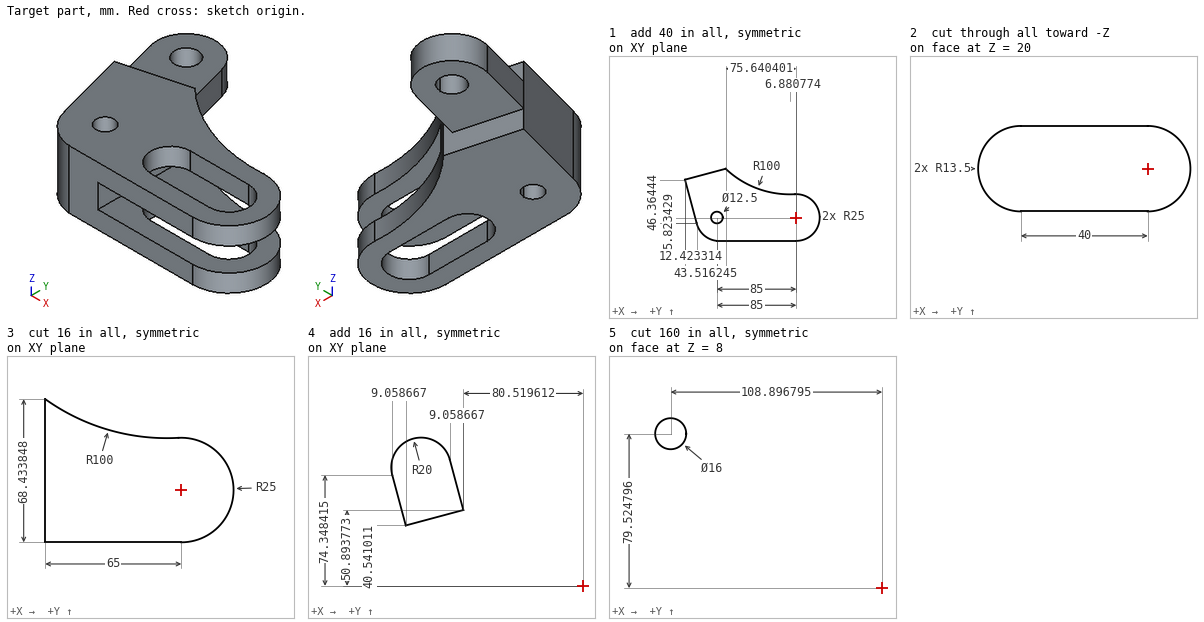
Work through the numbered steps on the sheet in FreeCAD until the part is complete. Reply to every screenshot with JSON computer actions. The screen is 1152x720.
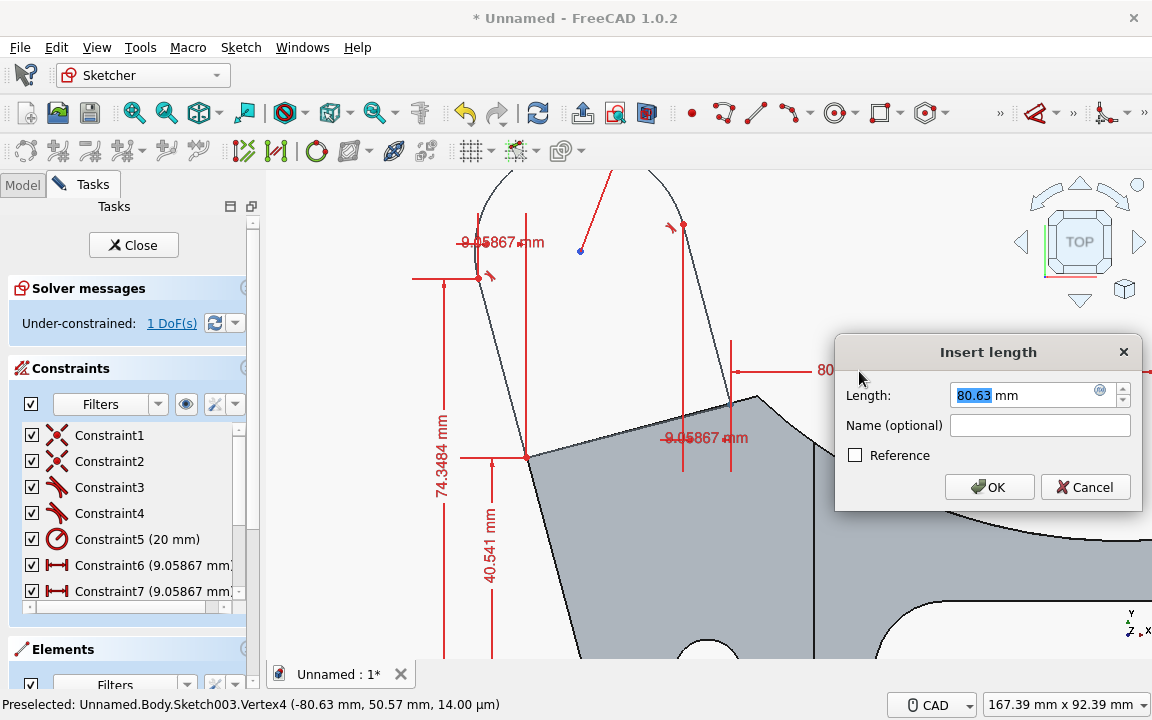
{"action": "type", "text": "80.519612"}
{"action": "key", "text": "Return"}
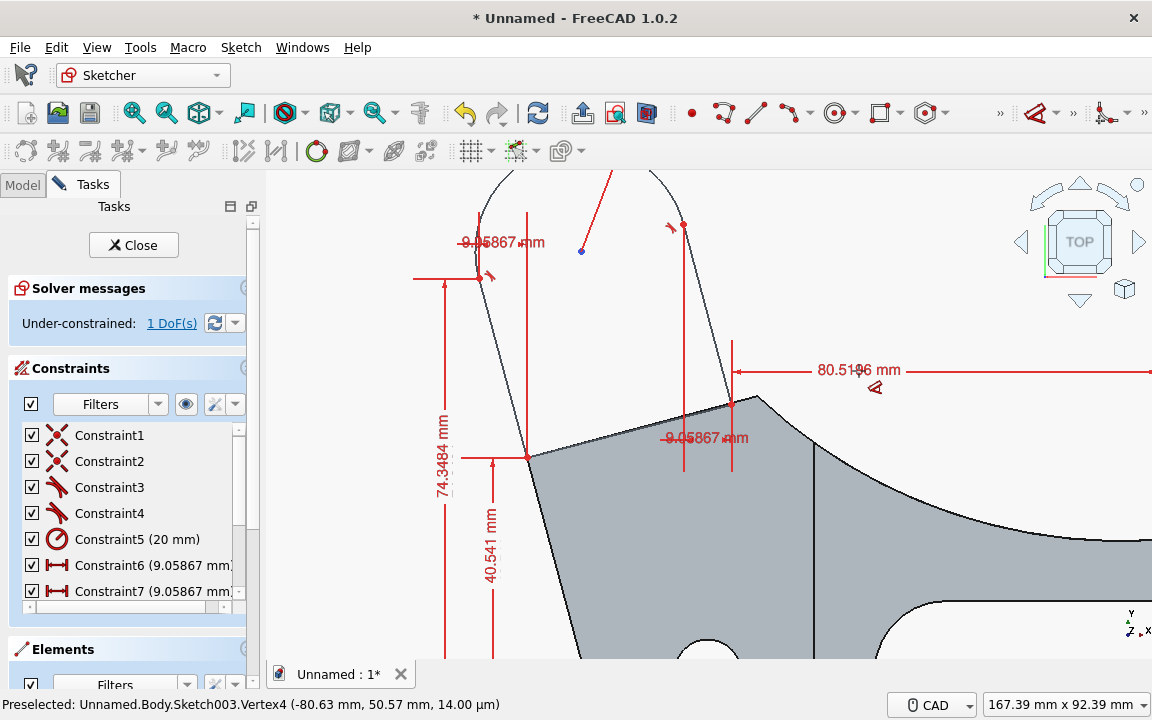
{"action": "left_click", "coordinate": [732, 405]}
{"action": "left_click", "coordinate": [698, 518]}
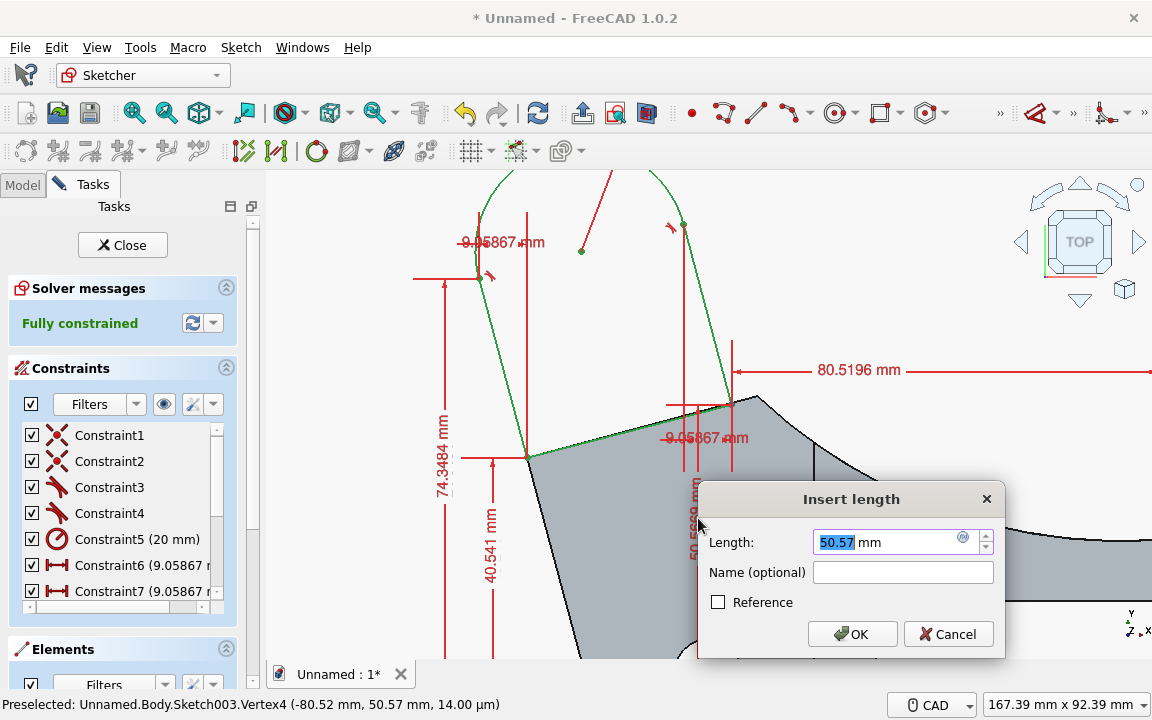
{"action": "type", "text": "50.893773"}
{"action": "key", "text": "Return"}
{"action": "key", "text": "Escape"}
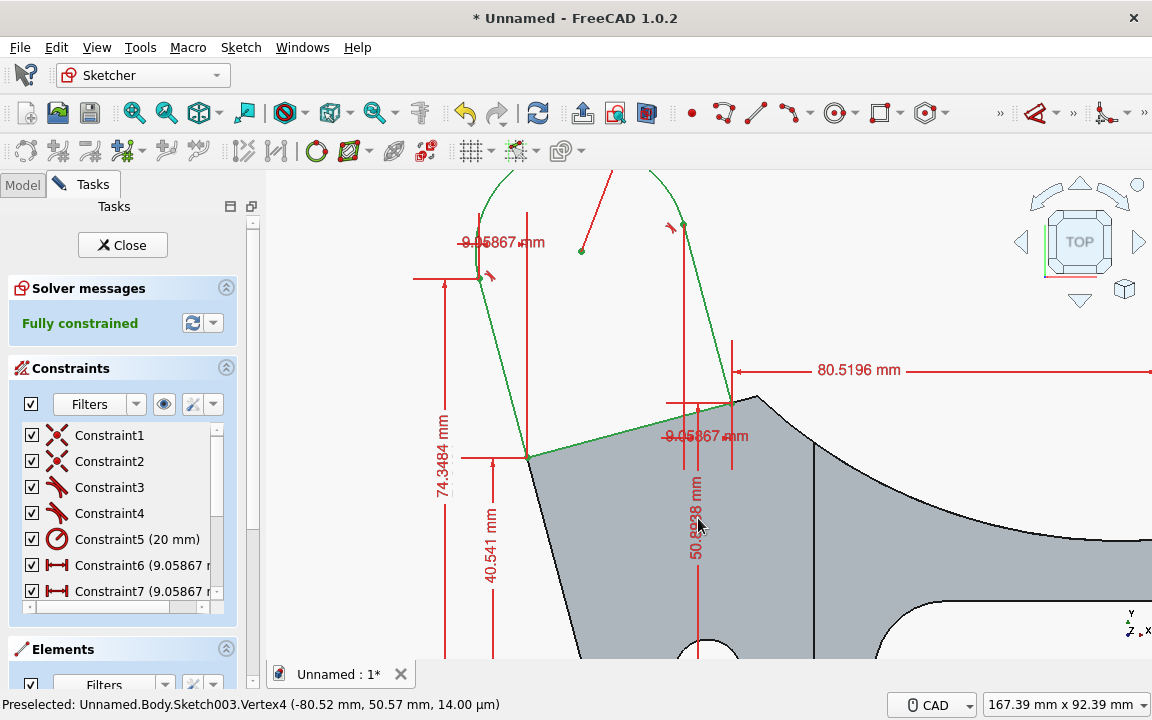
{"action": "left_click", "coordinate": [123, 245]}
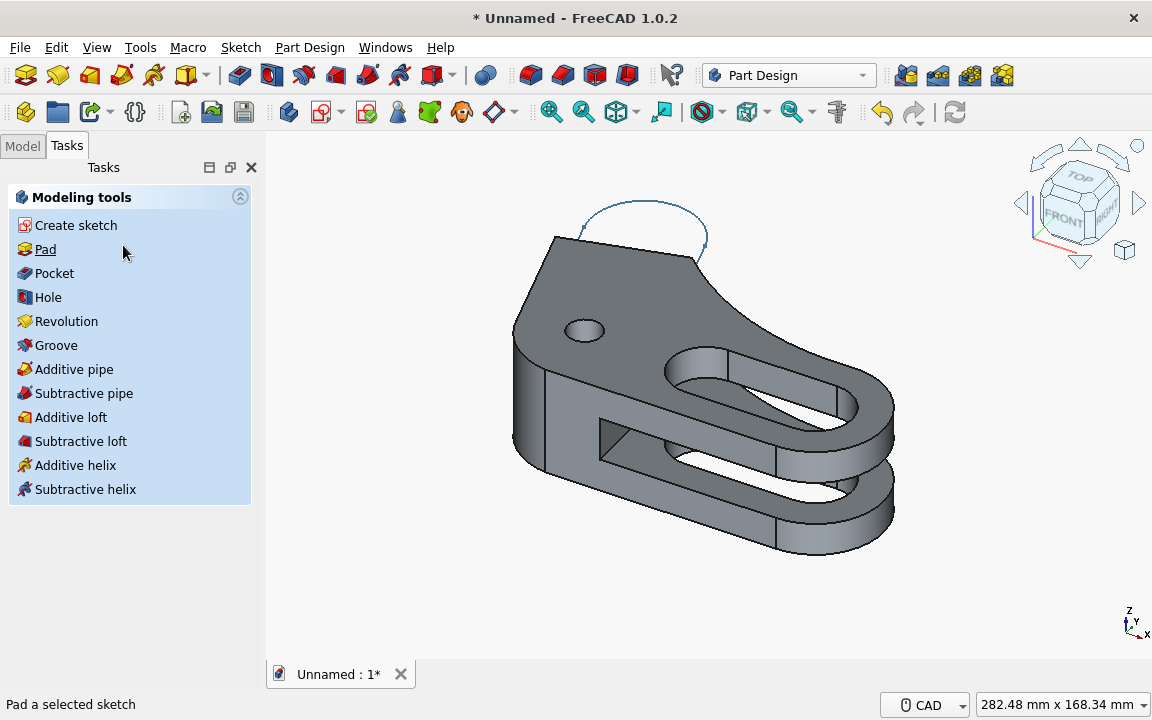
{"action": "left_click", "coordinate": [26, 76]}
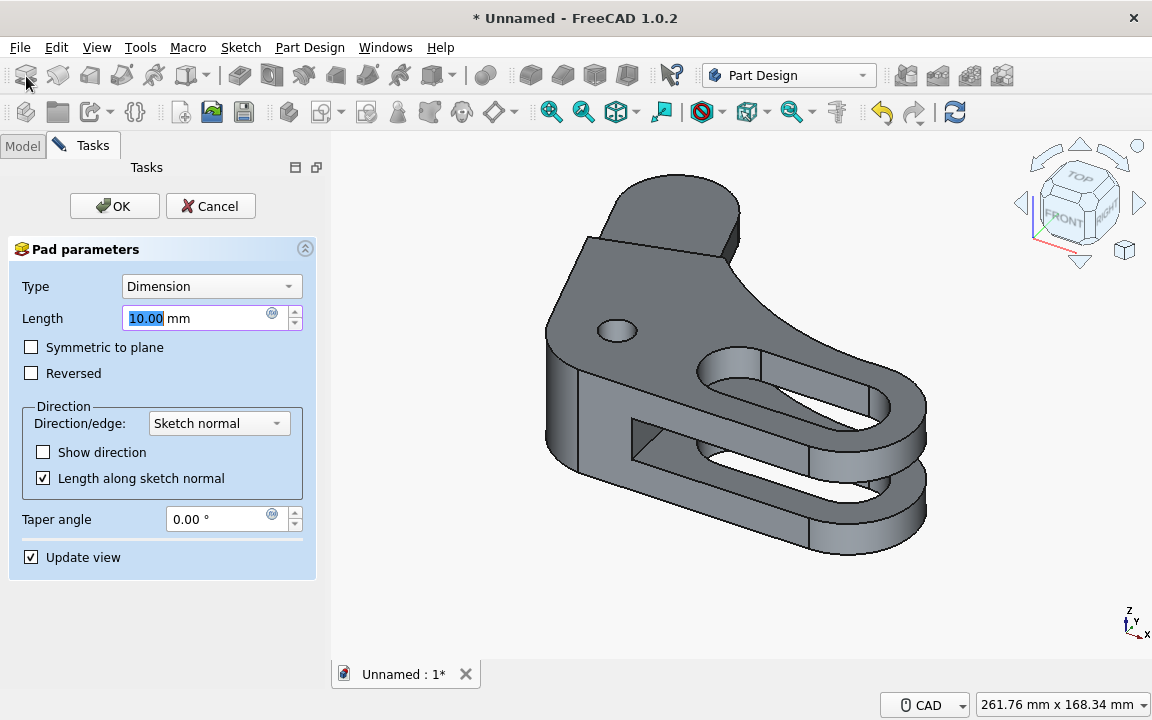
{"action": "type", "text": "16"}
{"action": "key", "text": "Tab"}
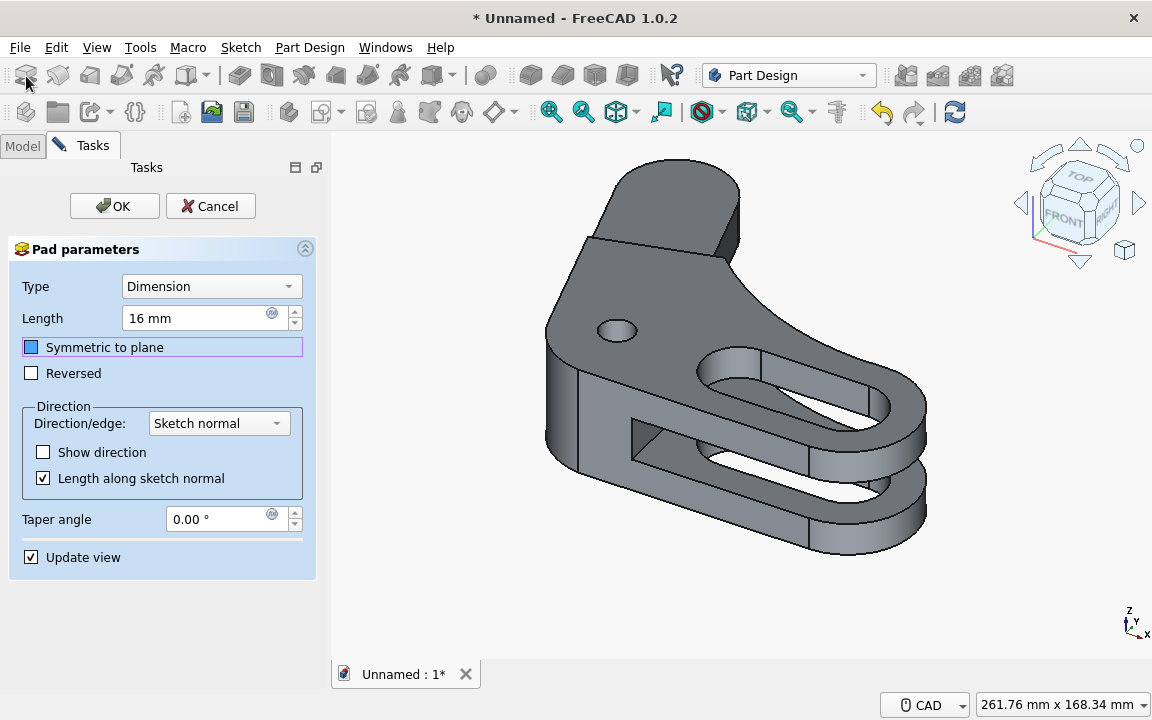
{"action": "left_click", "coordinate": [30, 347]}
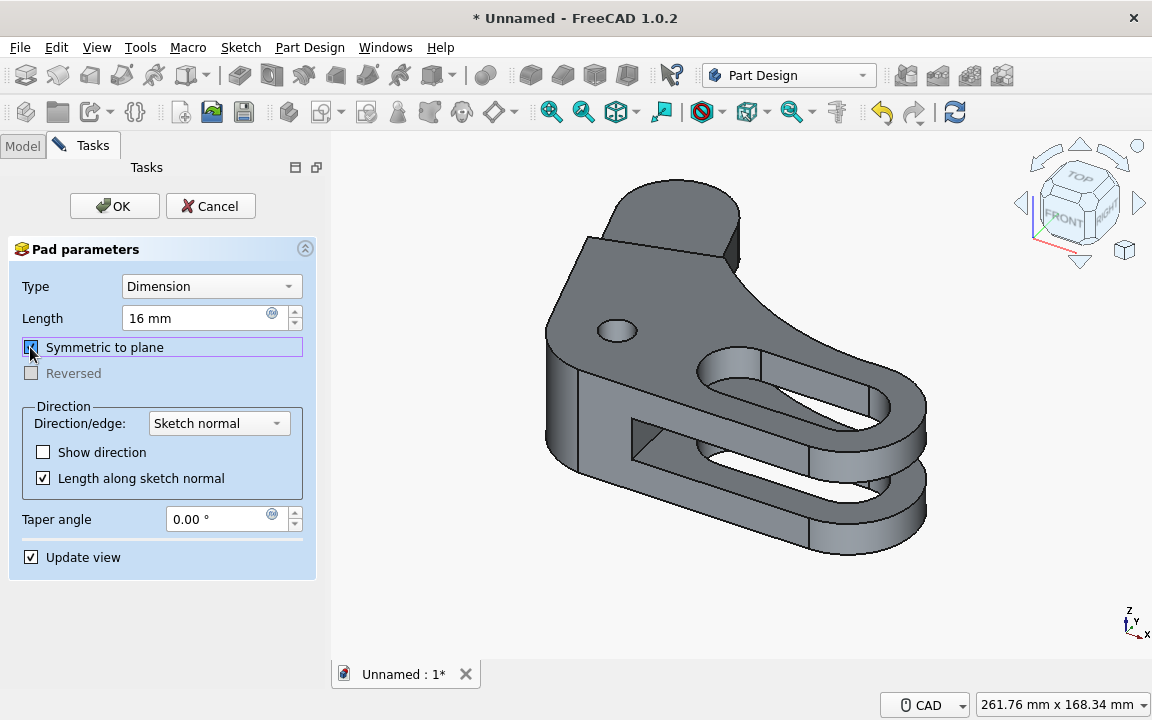
{"action": "left_click", "coordinate": [115, 206]}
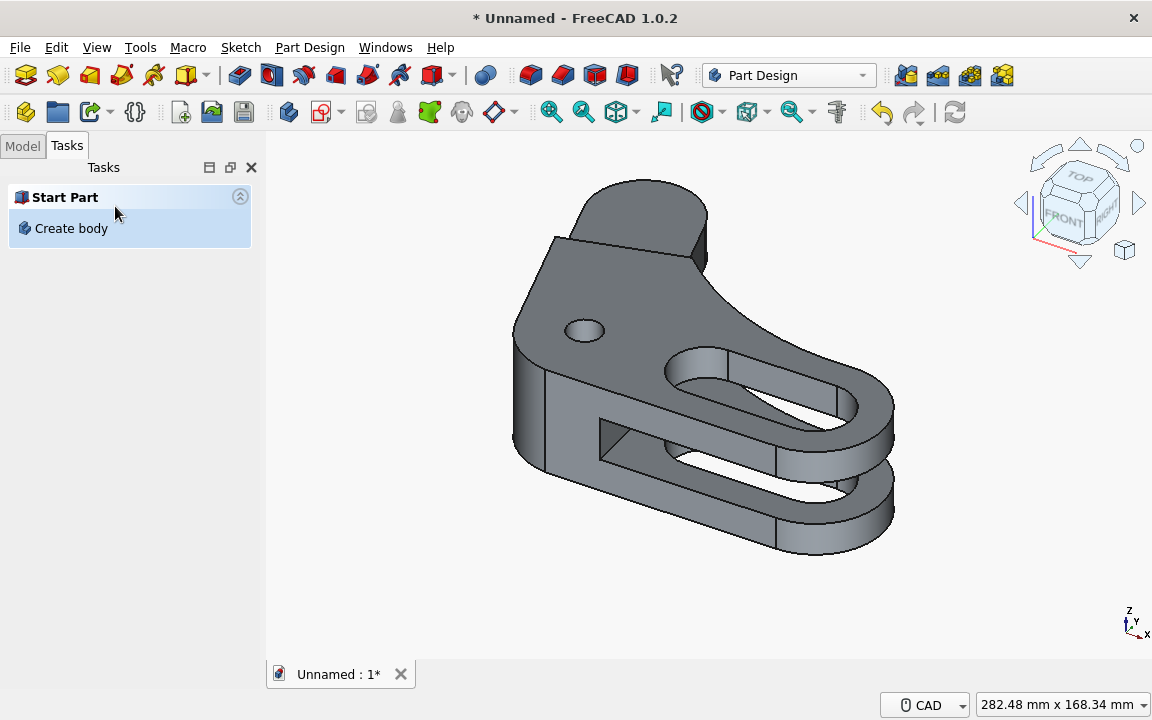
{"action": "left_click", "coordinate": [641, 234]}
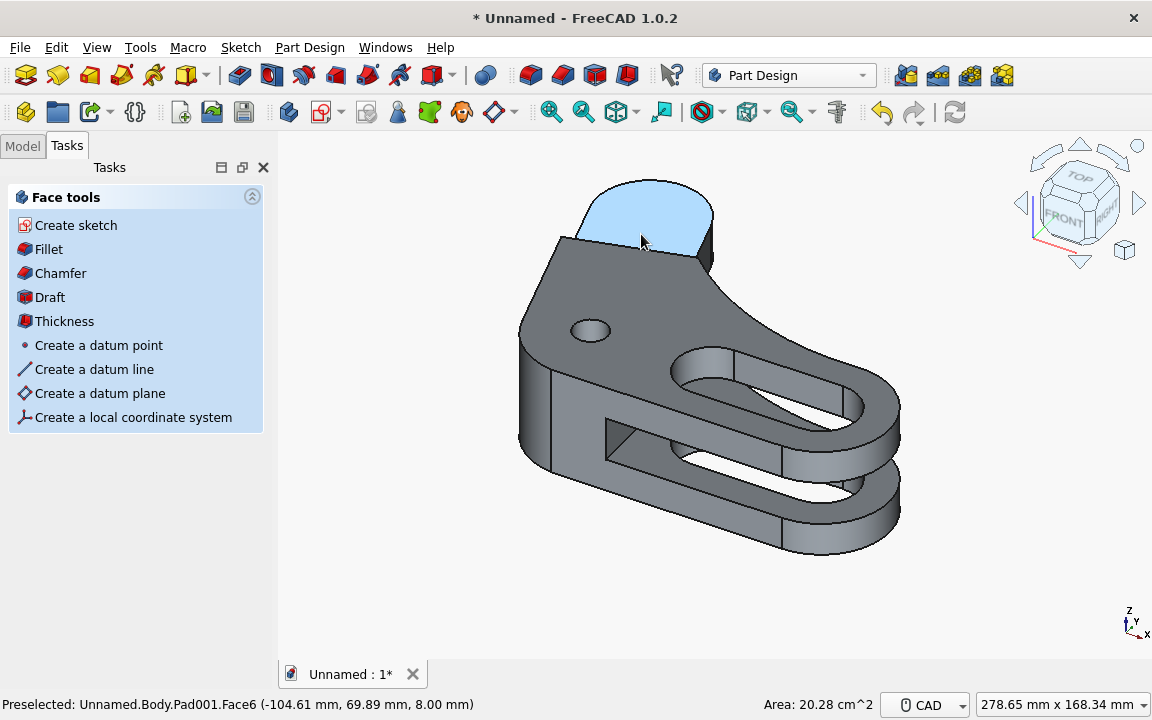
{"action": "left_click", "coordinate": [322, 112]}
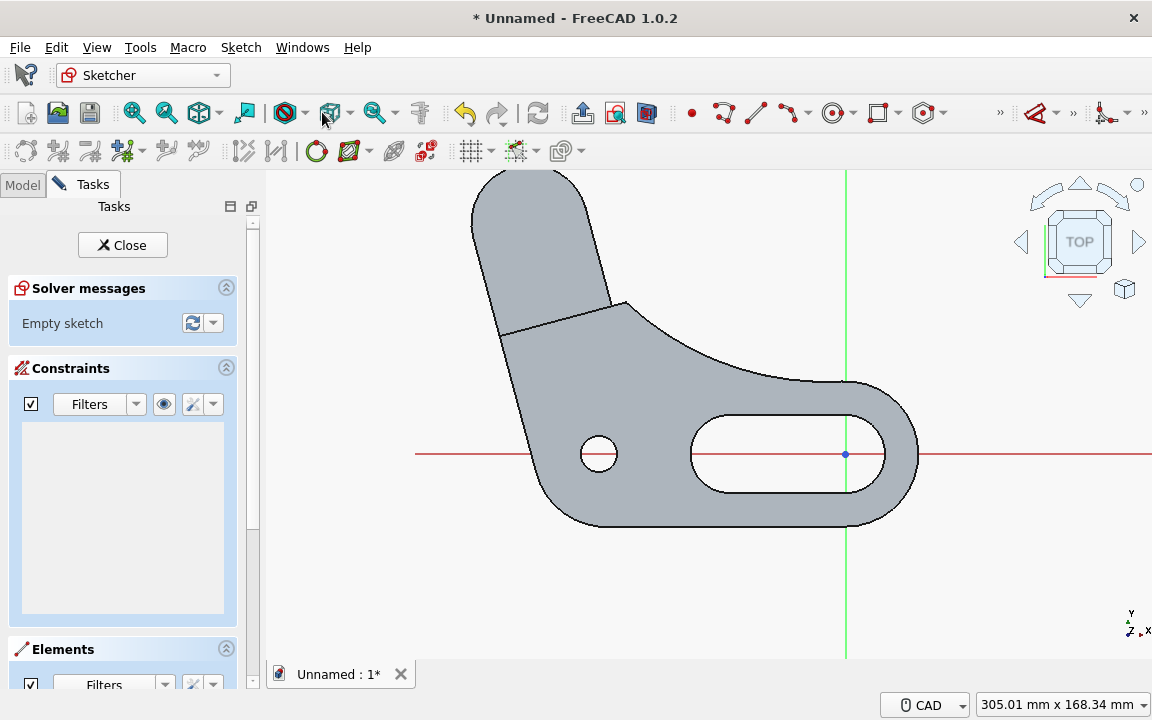
{"action": "scroll", "coordinate": [640, 414], "scroll_direction": "down", "scroll_amount": 5}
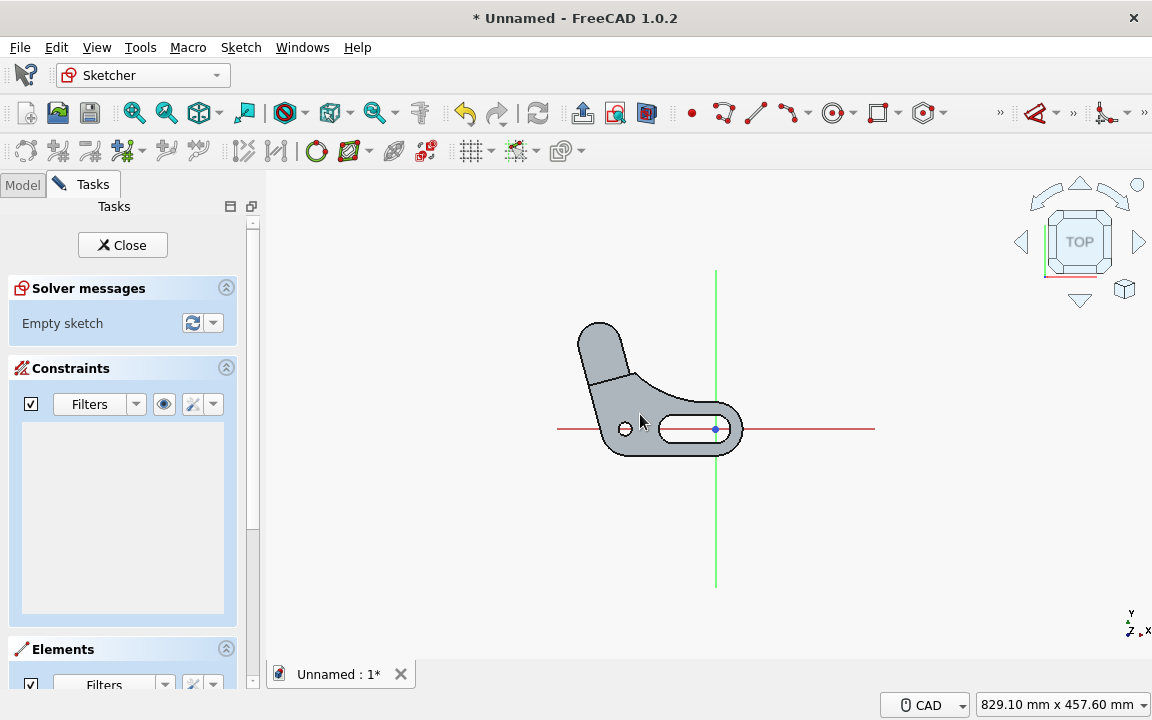
{"action": "scroll", "coordinate": [597, 339], "scroll_direction": "up", "scroll_amount": 14}